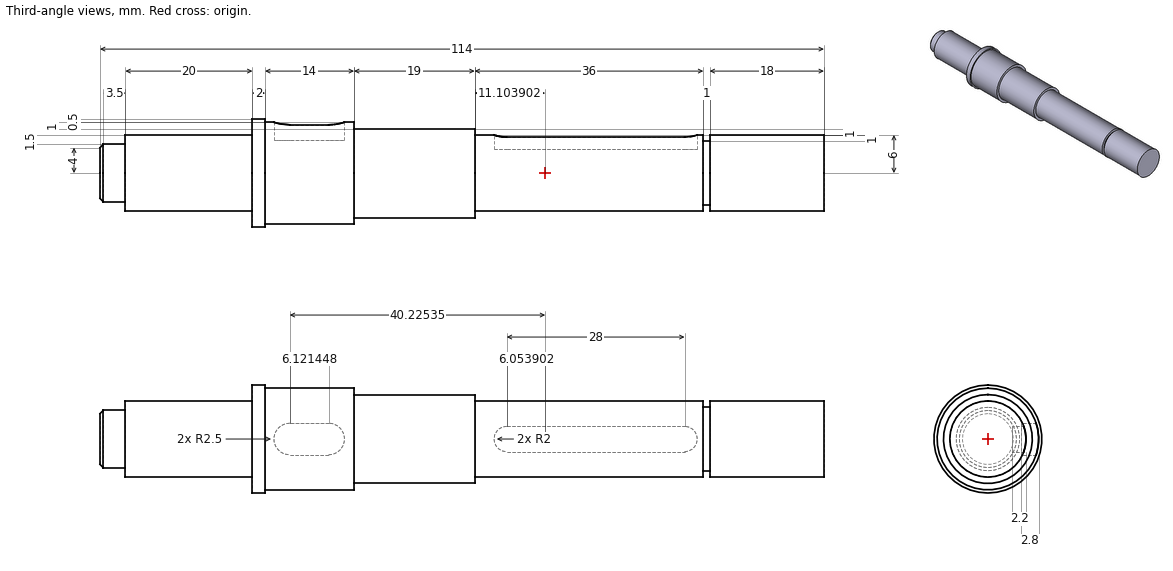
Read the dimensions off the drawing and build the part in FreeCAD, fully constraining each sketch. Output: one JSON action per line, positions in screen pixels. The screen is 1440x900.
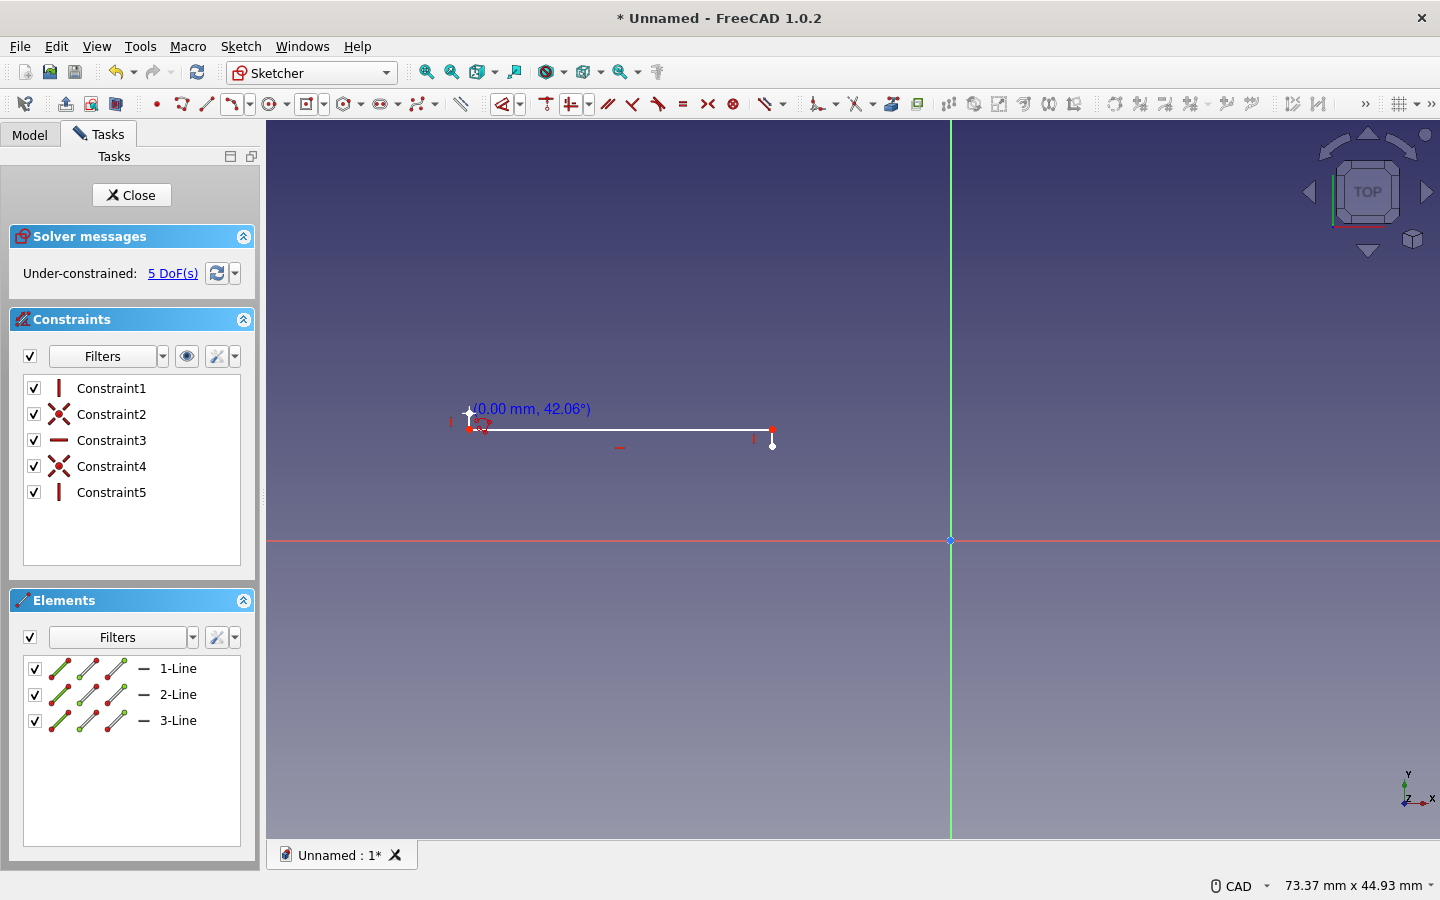
{"action": "scroll", "coordinate": [810, 483], "scroll_direction": "down", "scroll_amount": 5}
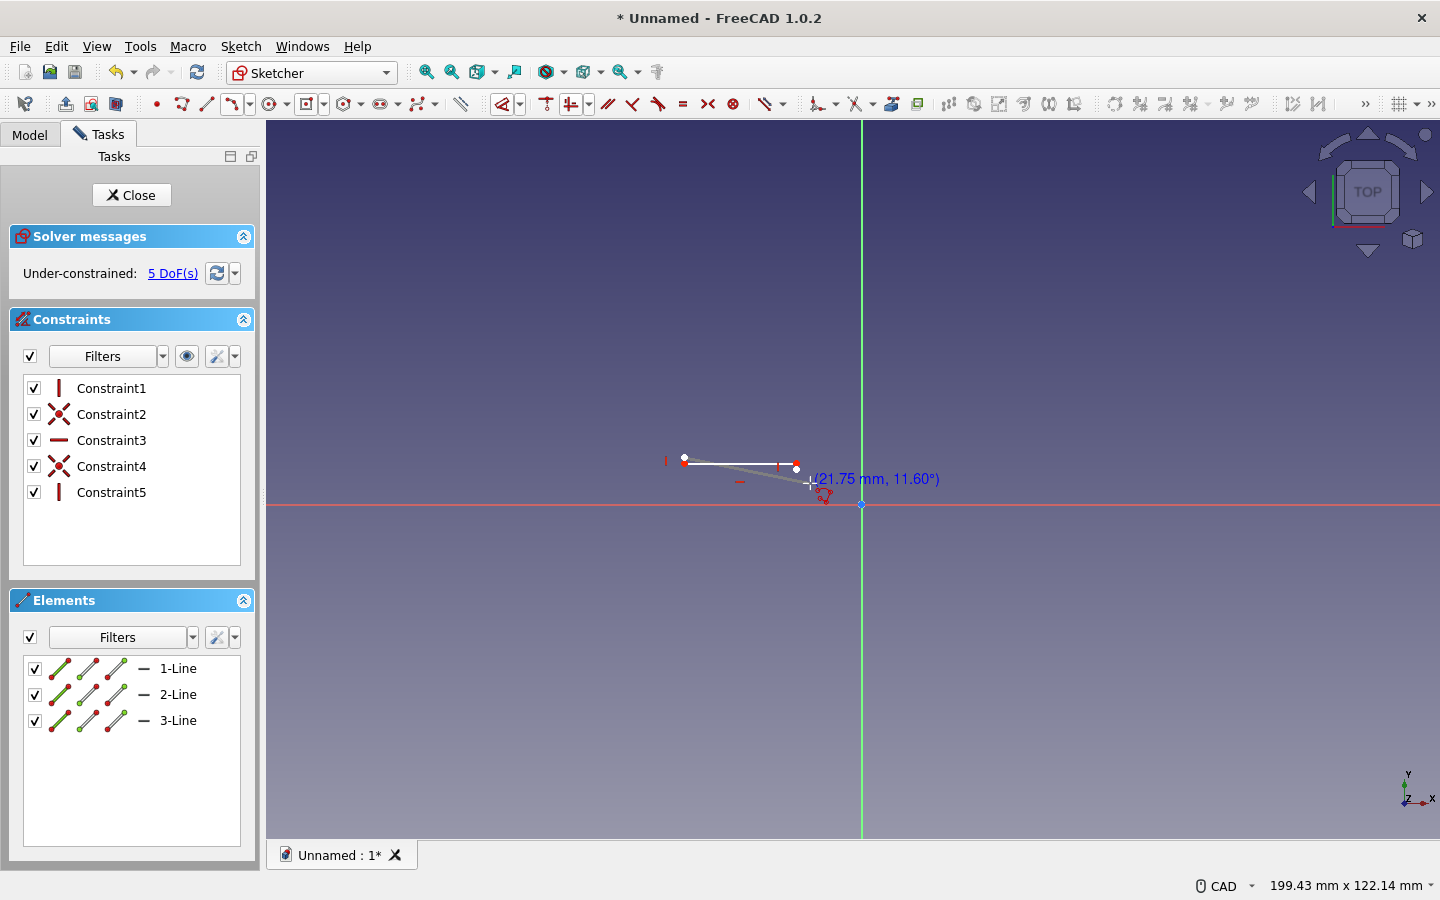
{"action": "left_click", "coordinate": [602, 458]}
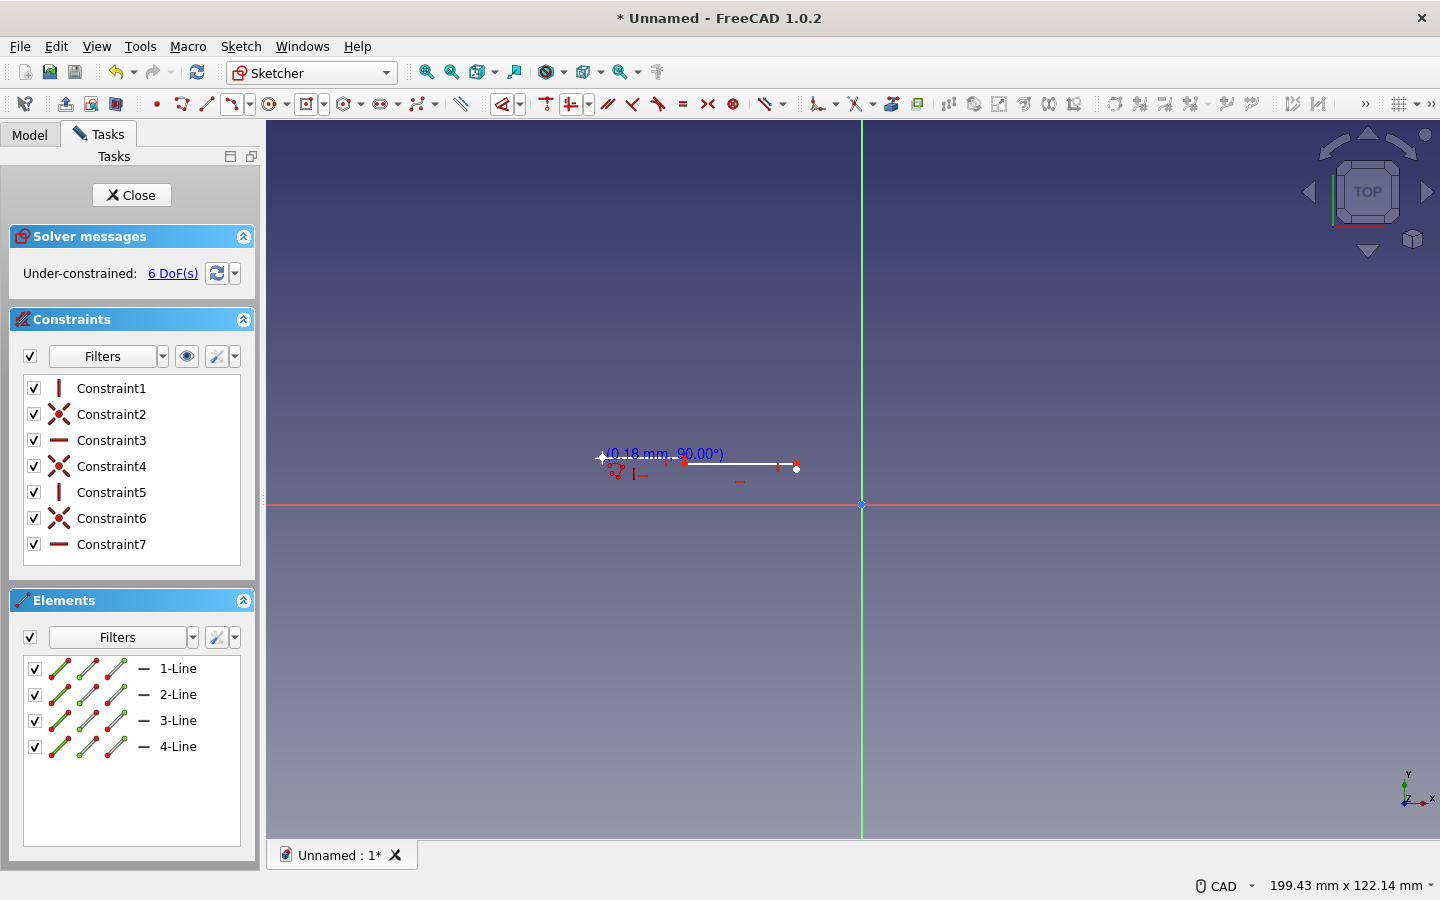
{"action": "scroll", "coordinate": [602, 455], "scroll_direction": "up", "scroll_amount": 9}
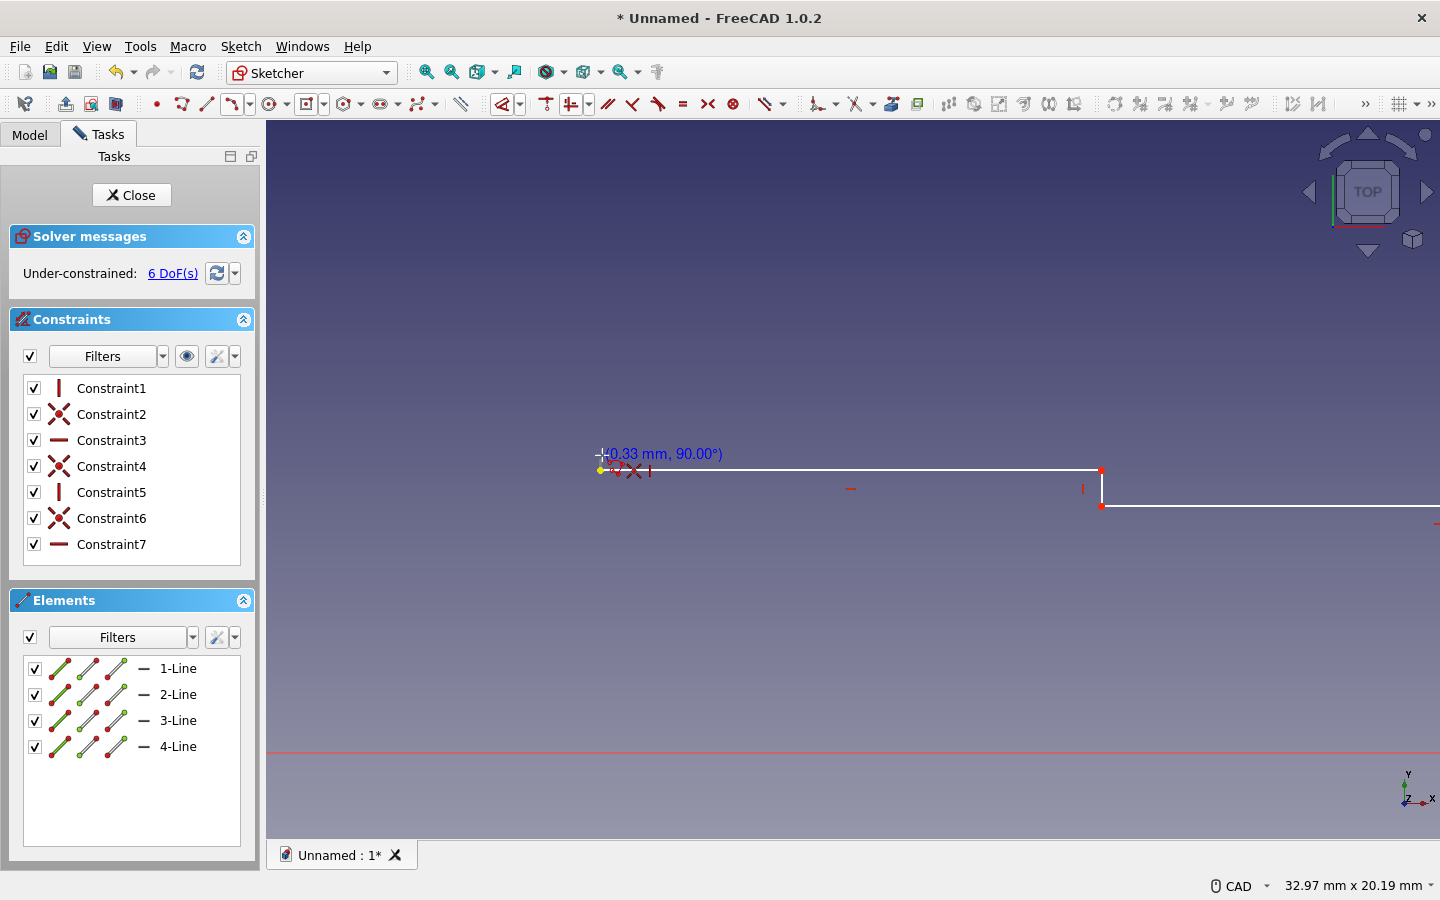
{"action": "left_click", "coordinate": [601, 450]}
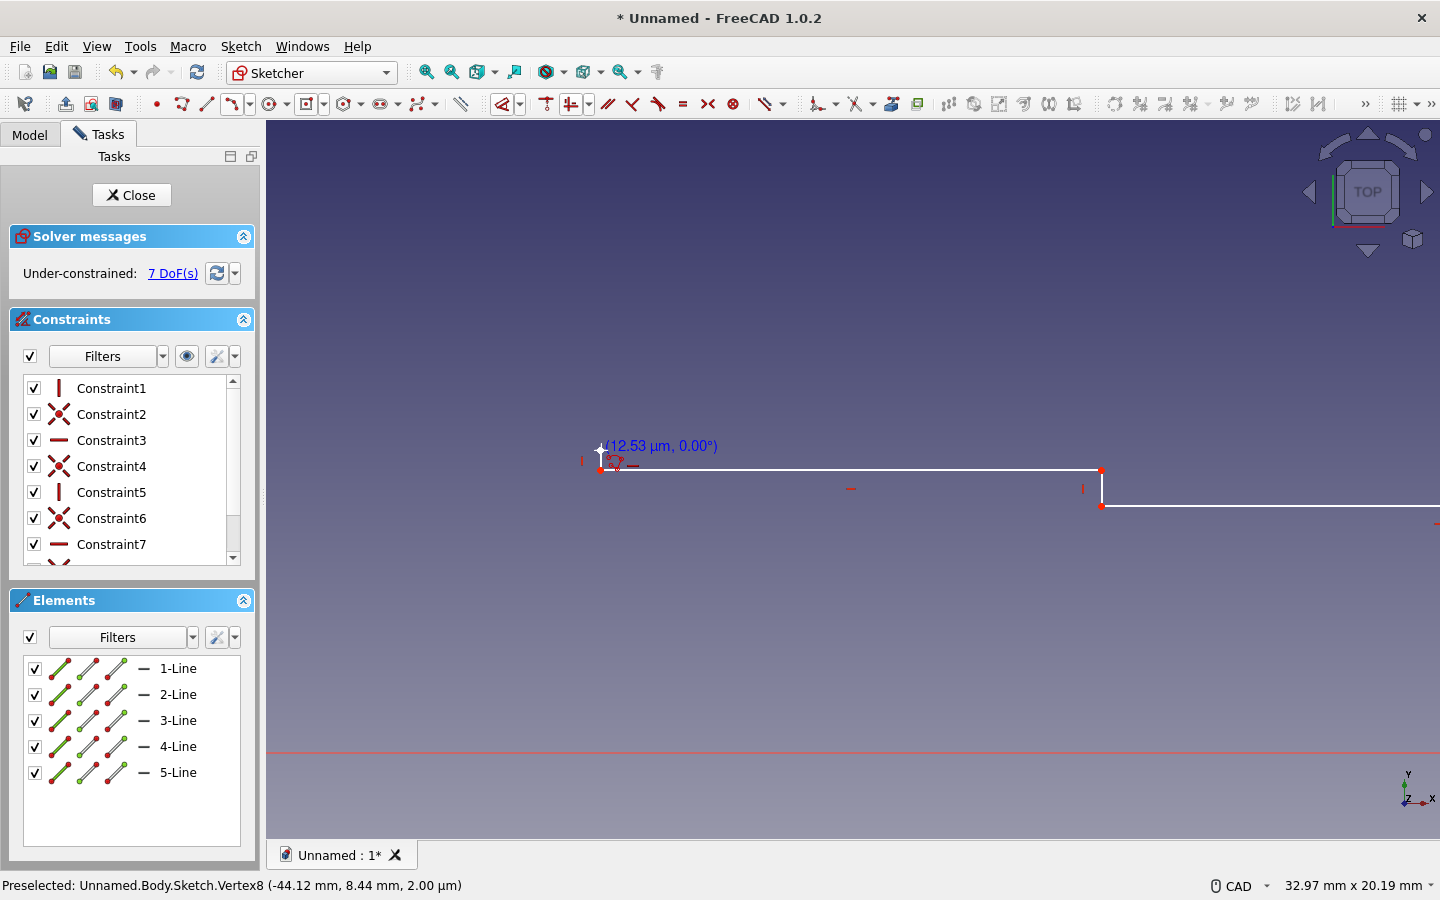
{"action": "scroll", "coordinate": [602, 455], "scroll_direction": "down", "scroll_amount": 9}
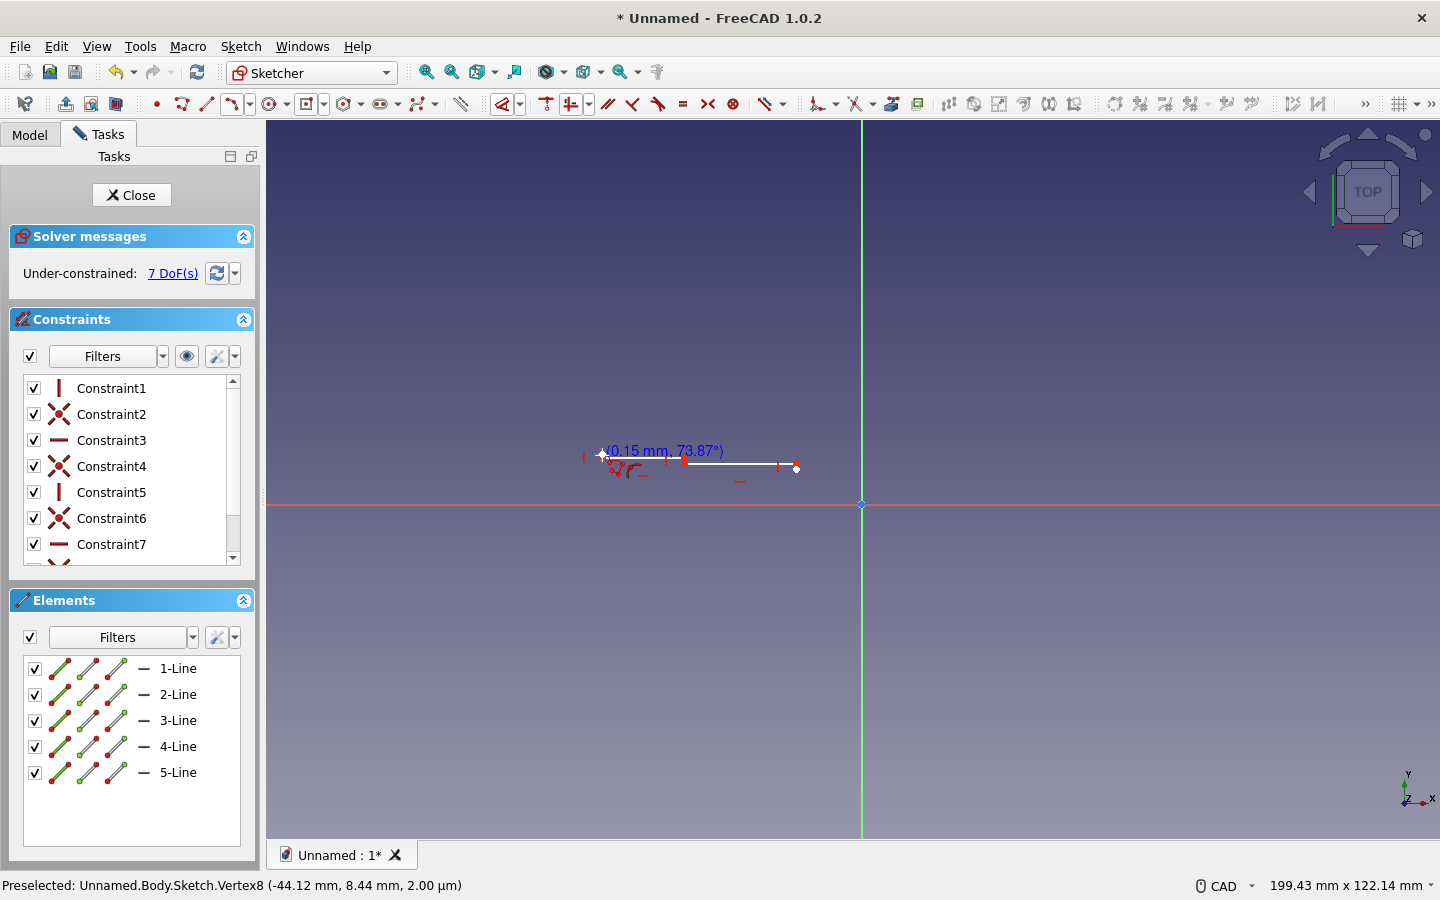
{"action": "scroll", "coordinate": [591, 455], "scroll_direction": "up", "scroll_amount": 2}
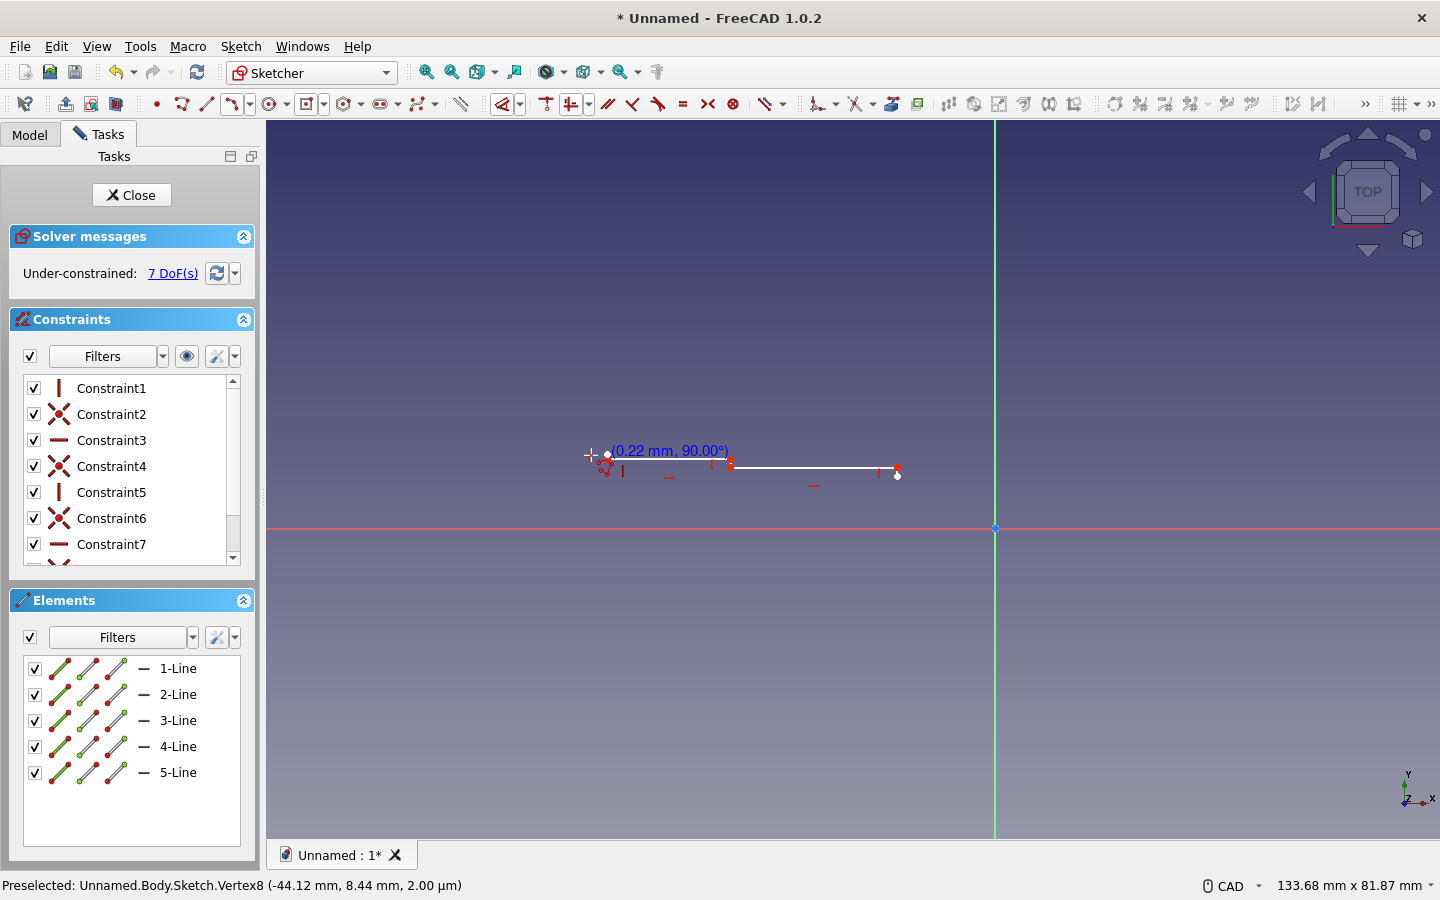
{"action": "left_click", "coordinate": [590, 454]}
{"action": "left_click", "coordinate": [590, 476]}
{"action": "left_click", "coordinate": [415, 476]}
{"action": "left_click", "coordinate": [415, 489]}
{"action": "left_click", "coordinate": [384, 489]}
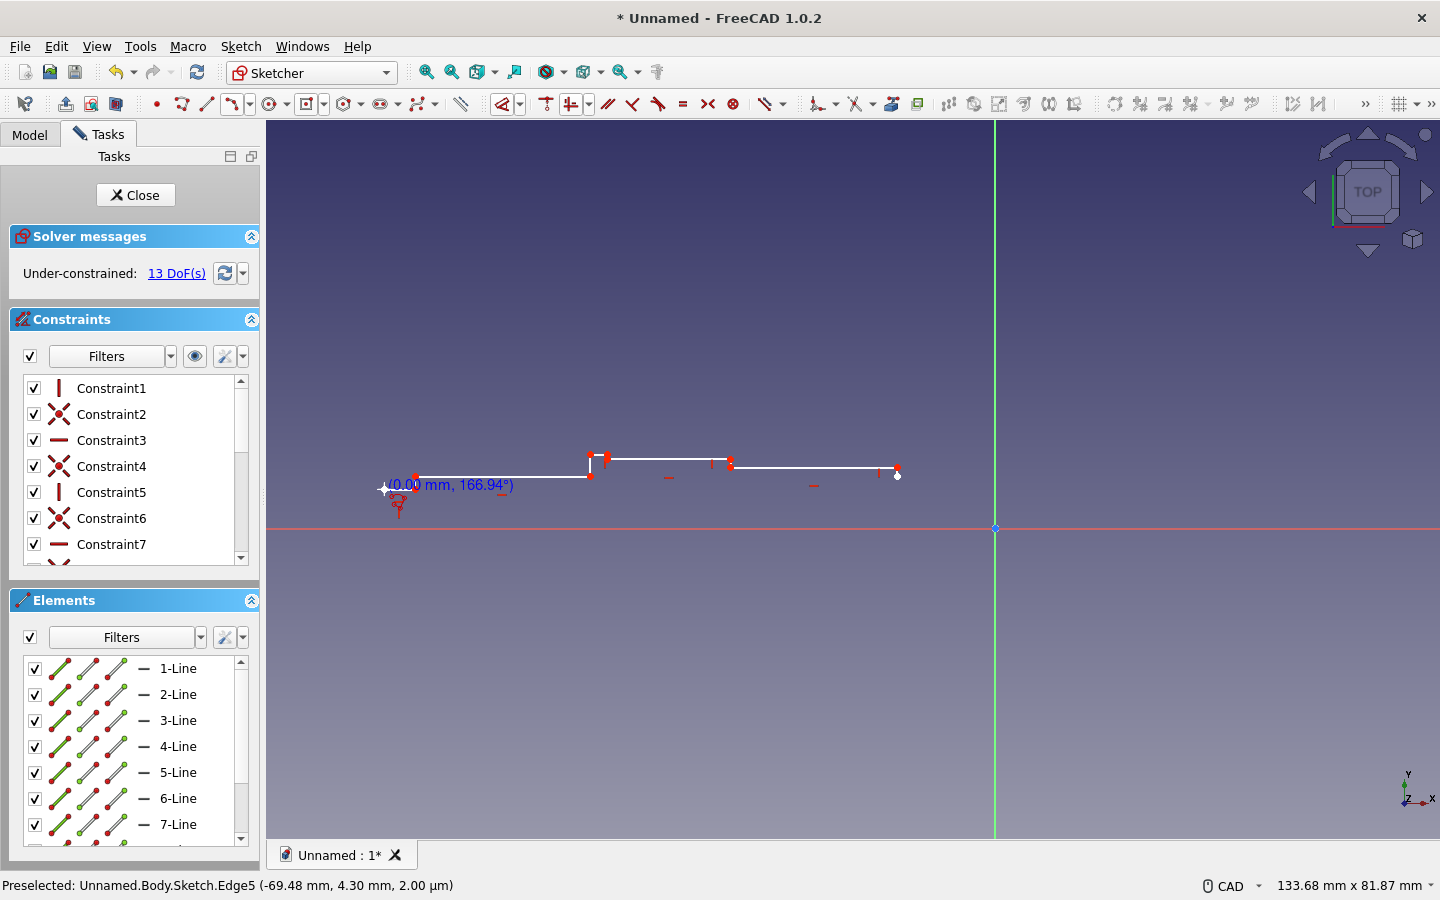
{"action": "scroll", "coordinate": [379, 494], "scroll_direction": "up", "scroll_amount": 5}